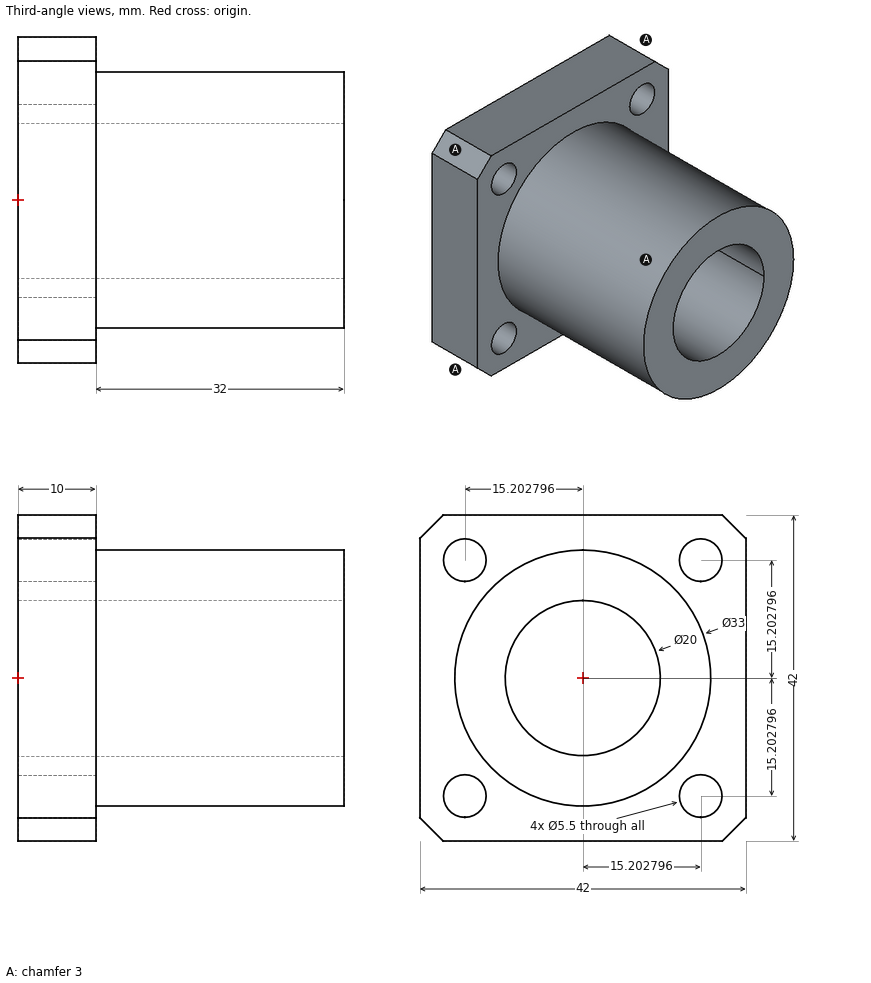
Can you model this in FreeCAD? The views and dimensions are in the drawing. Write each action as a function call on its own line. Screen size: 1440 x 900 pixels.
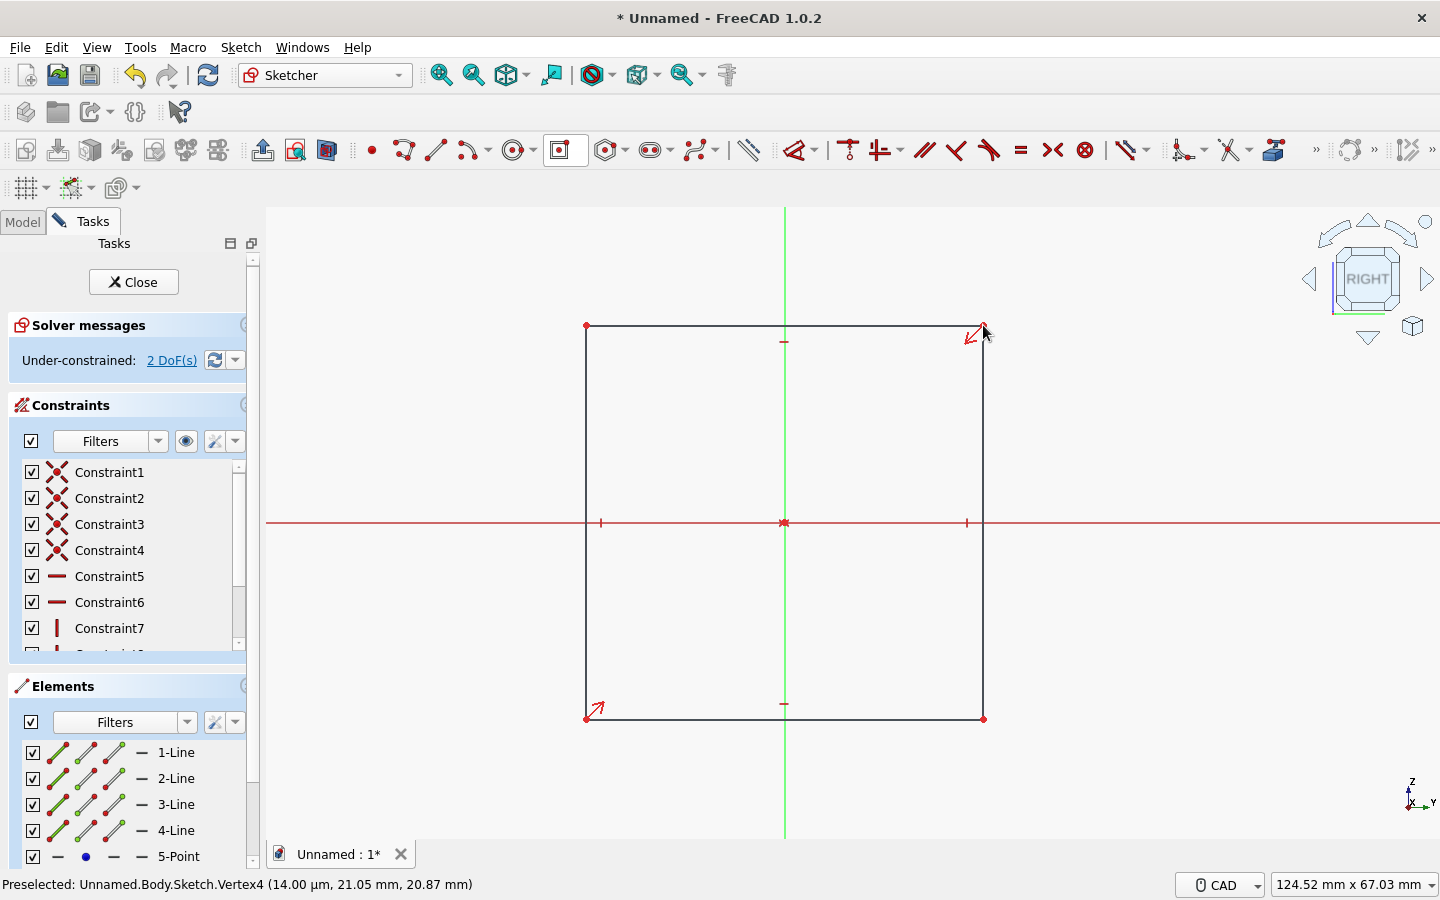
click(794, 150)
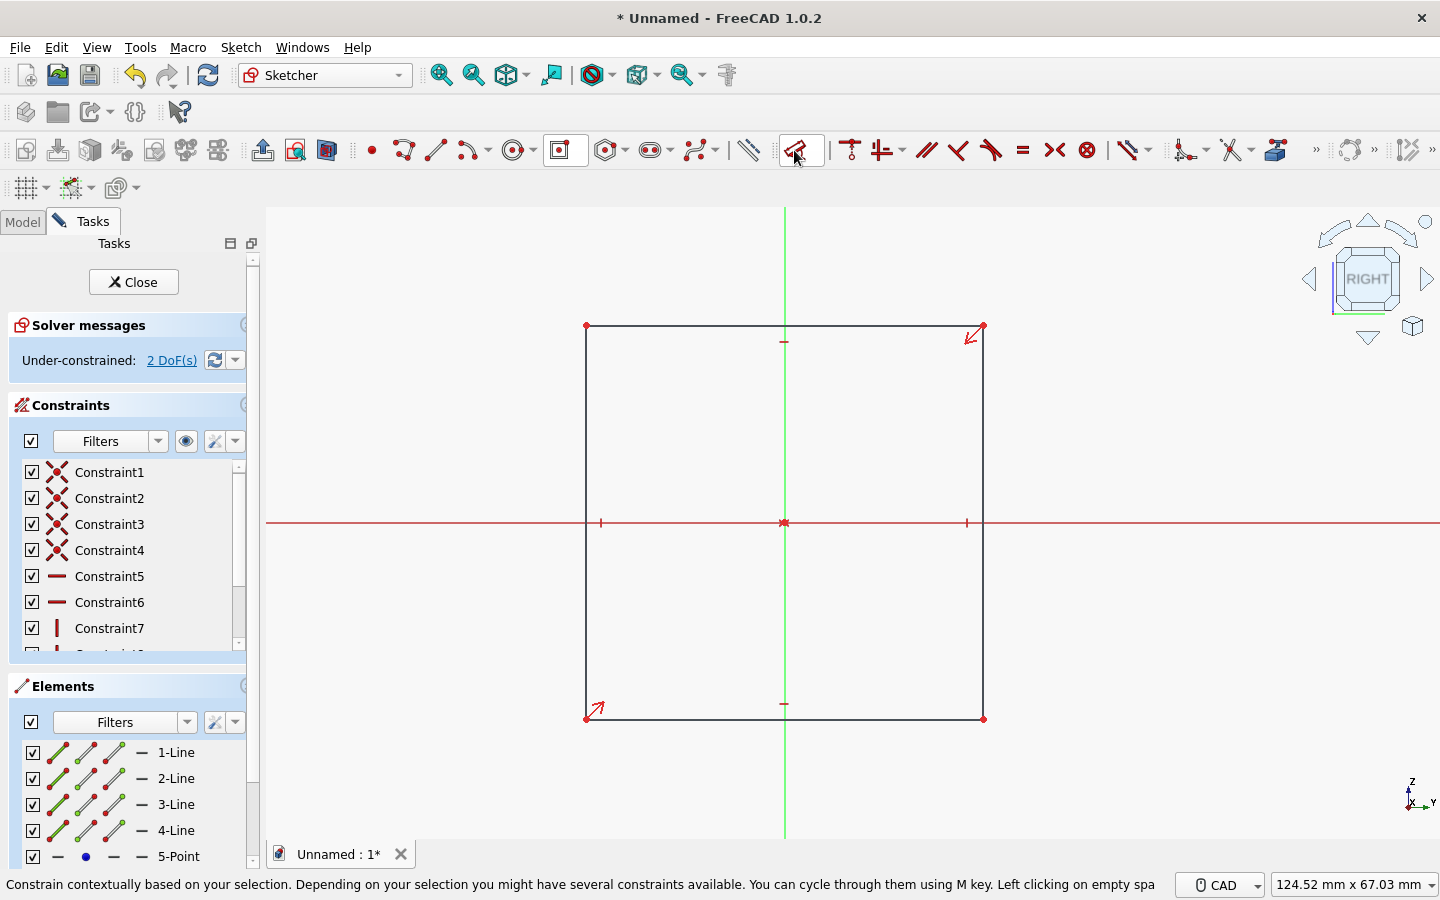
click(705, 720)
click(693, 754)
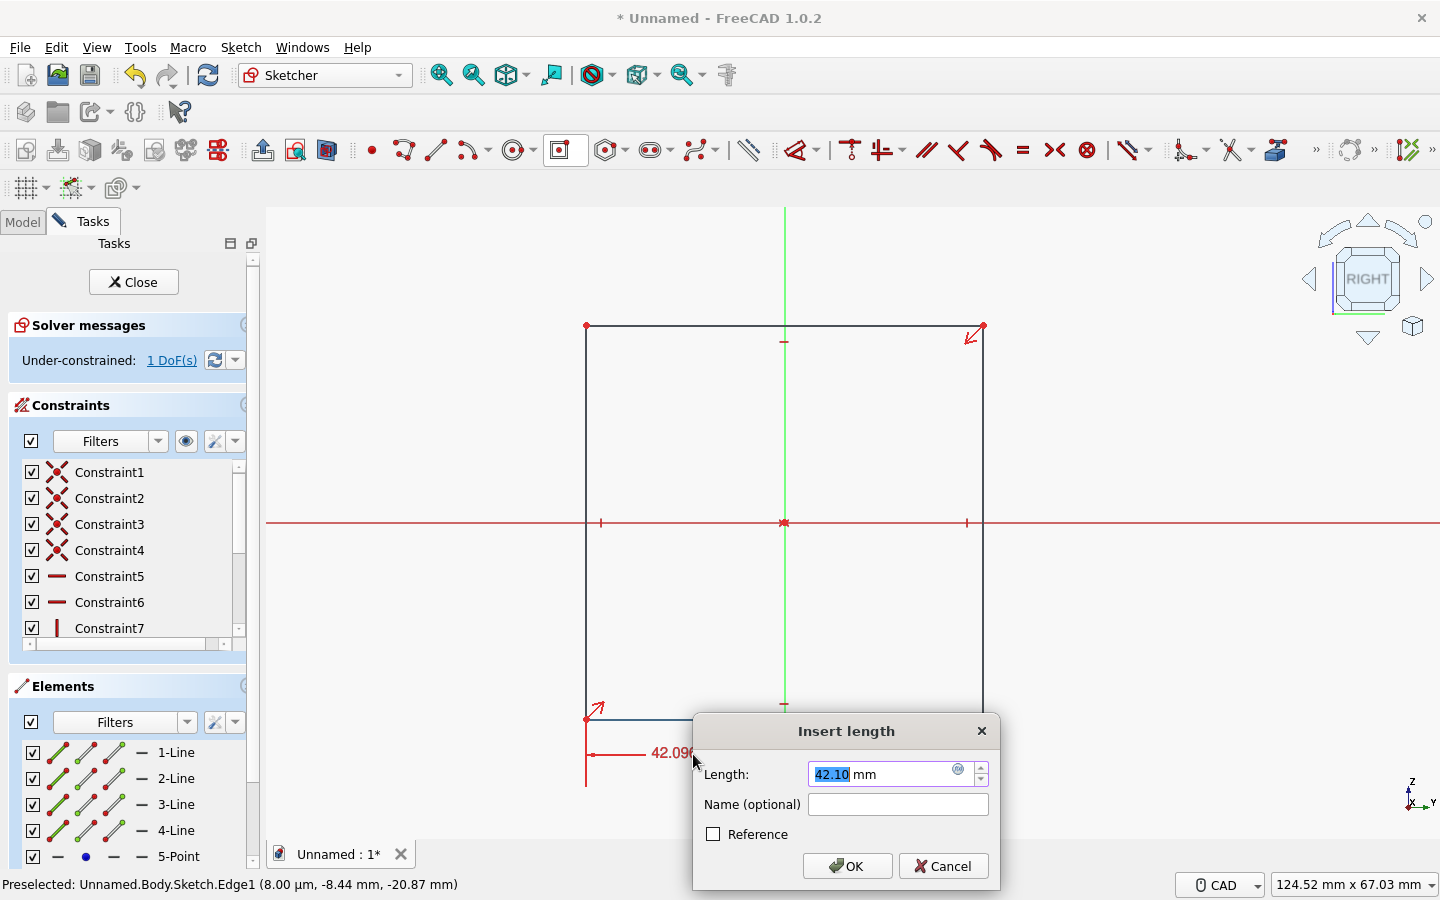
text(42)
key(Return)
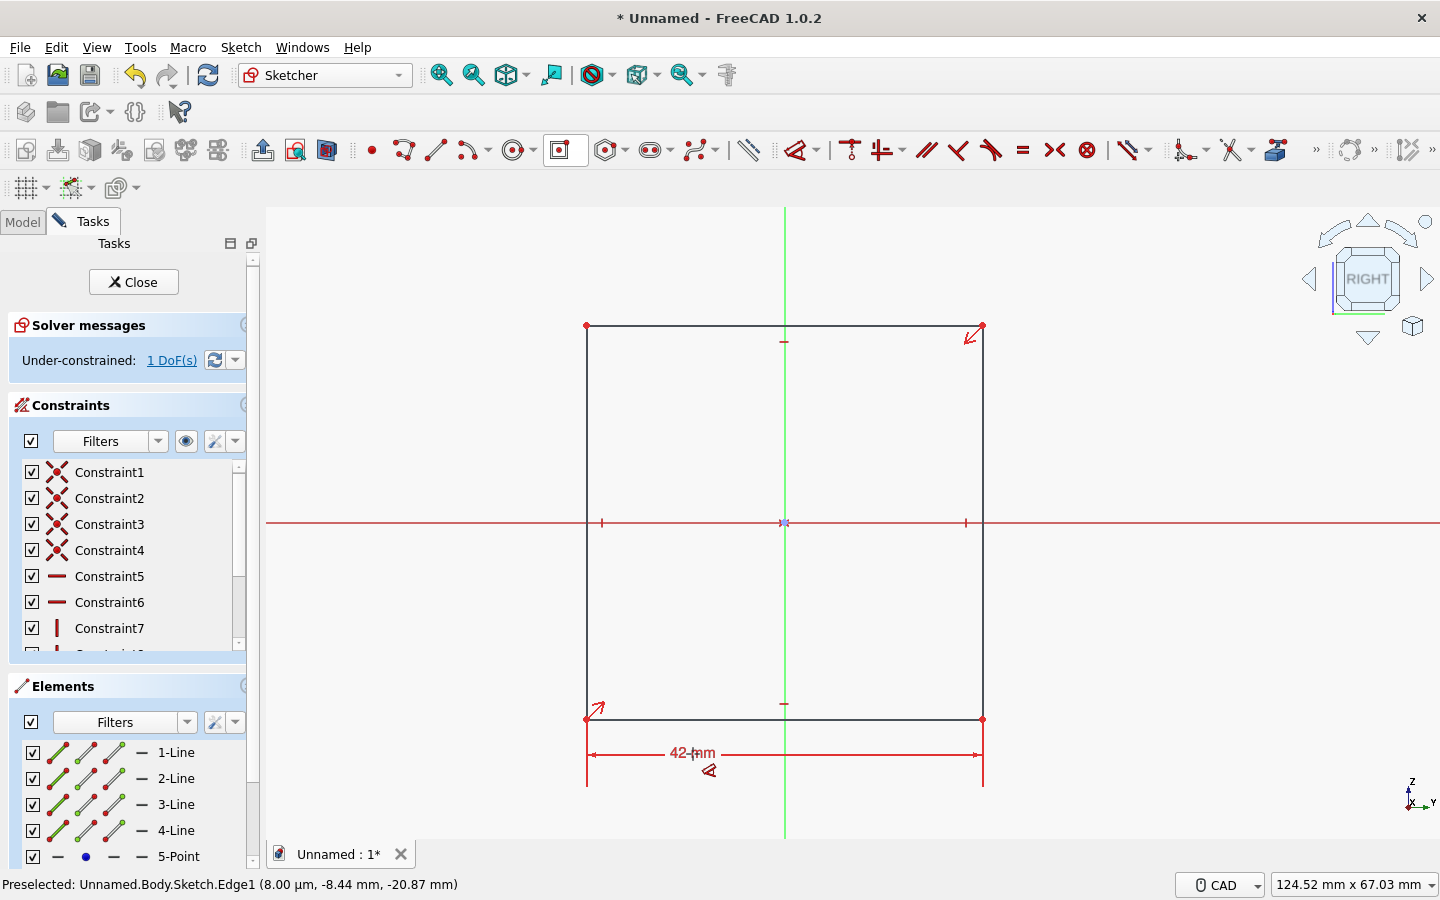
click(983, 601)
click(1017, 432)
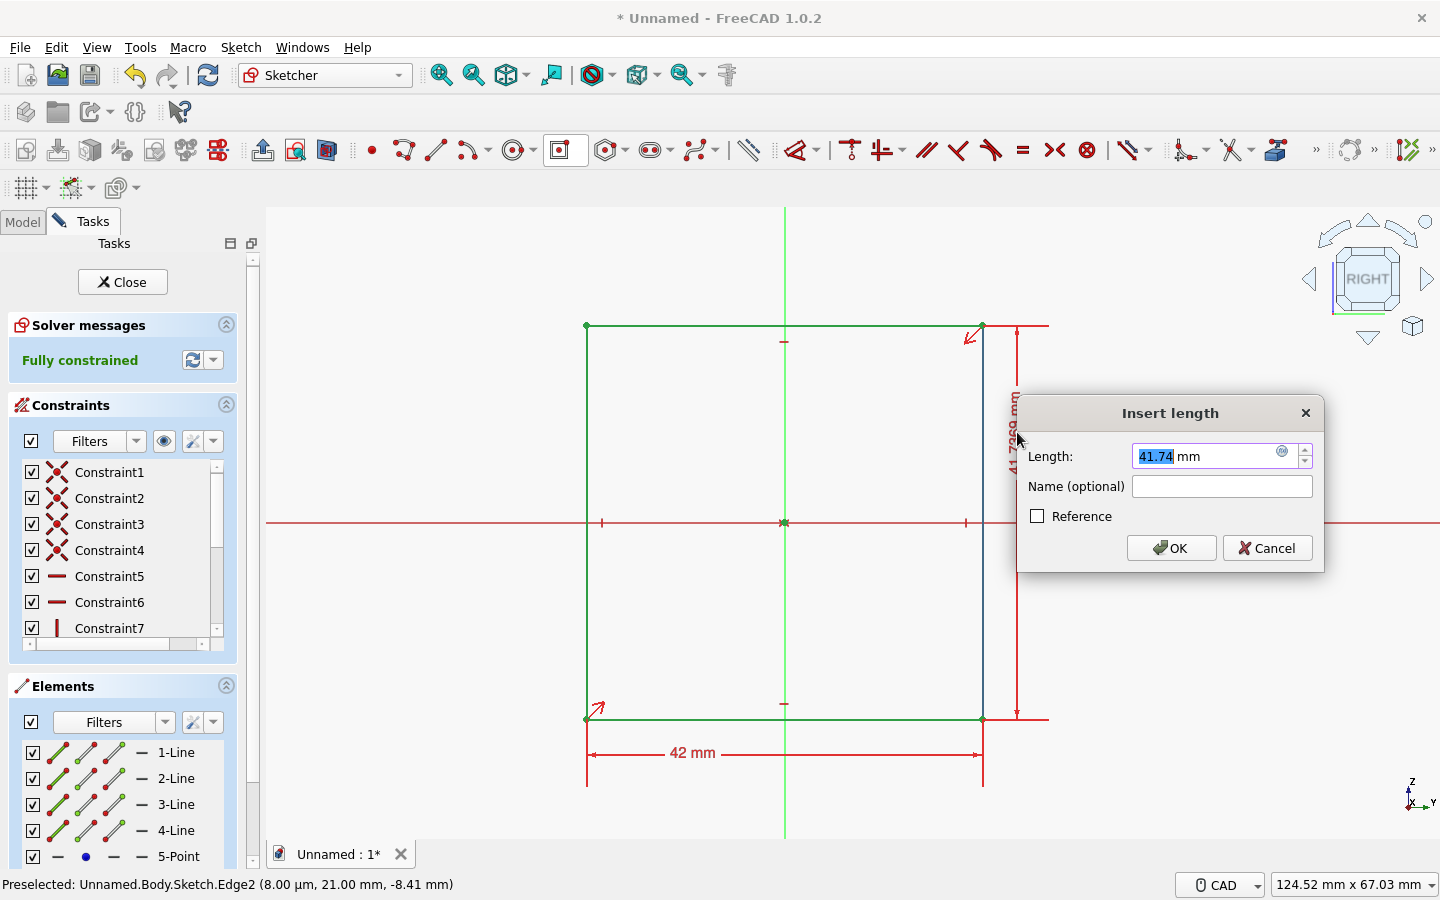
text(42)
key(Return)
key(Escape)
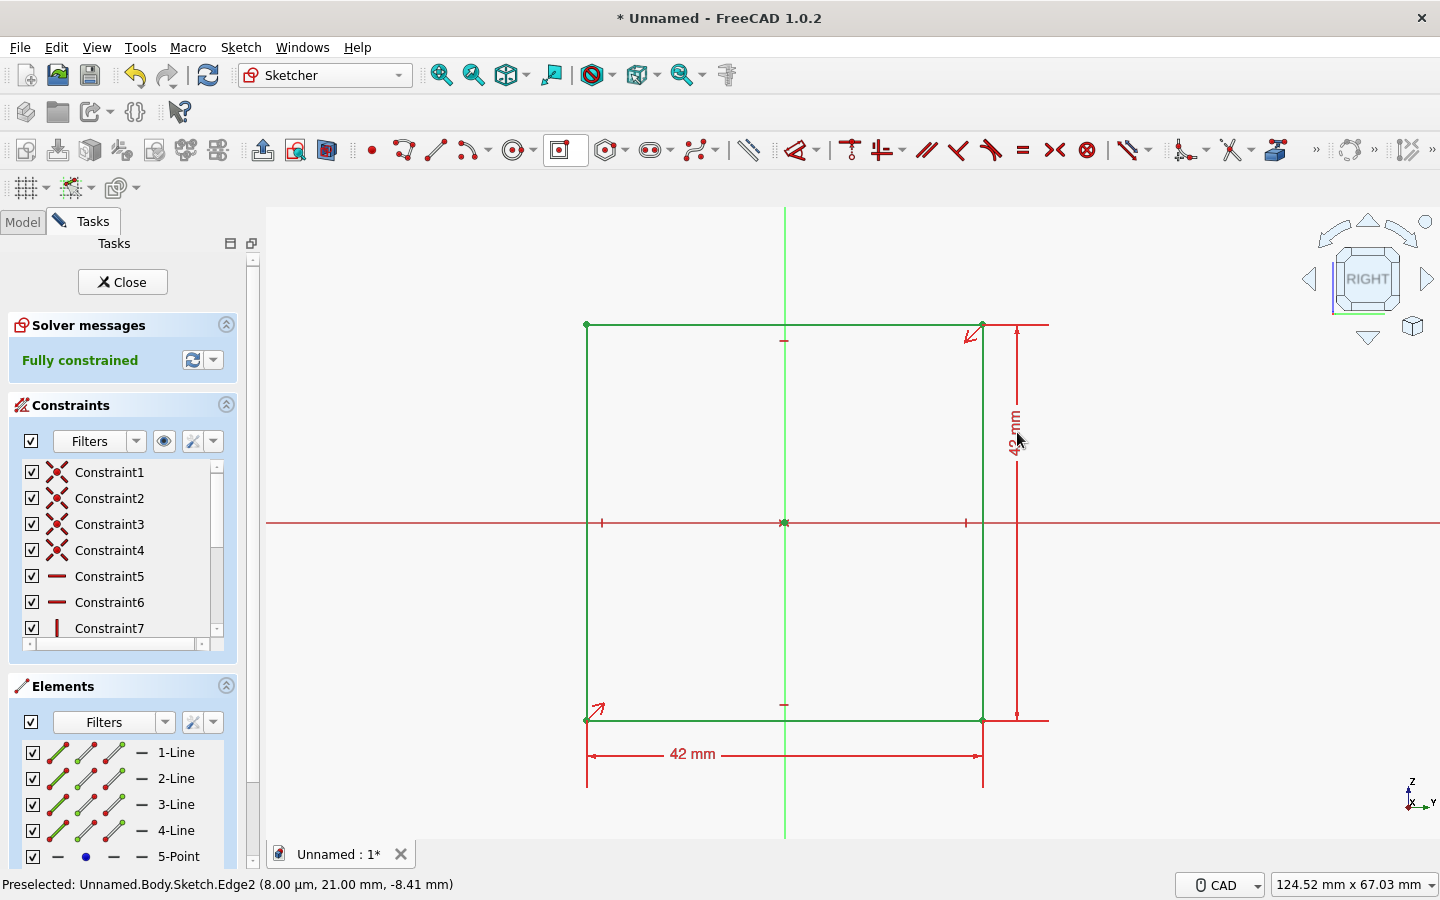
click(123, 282)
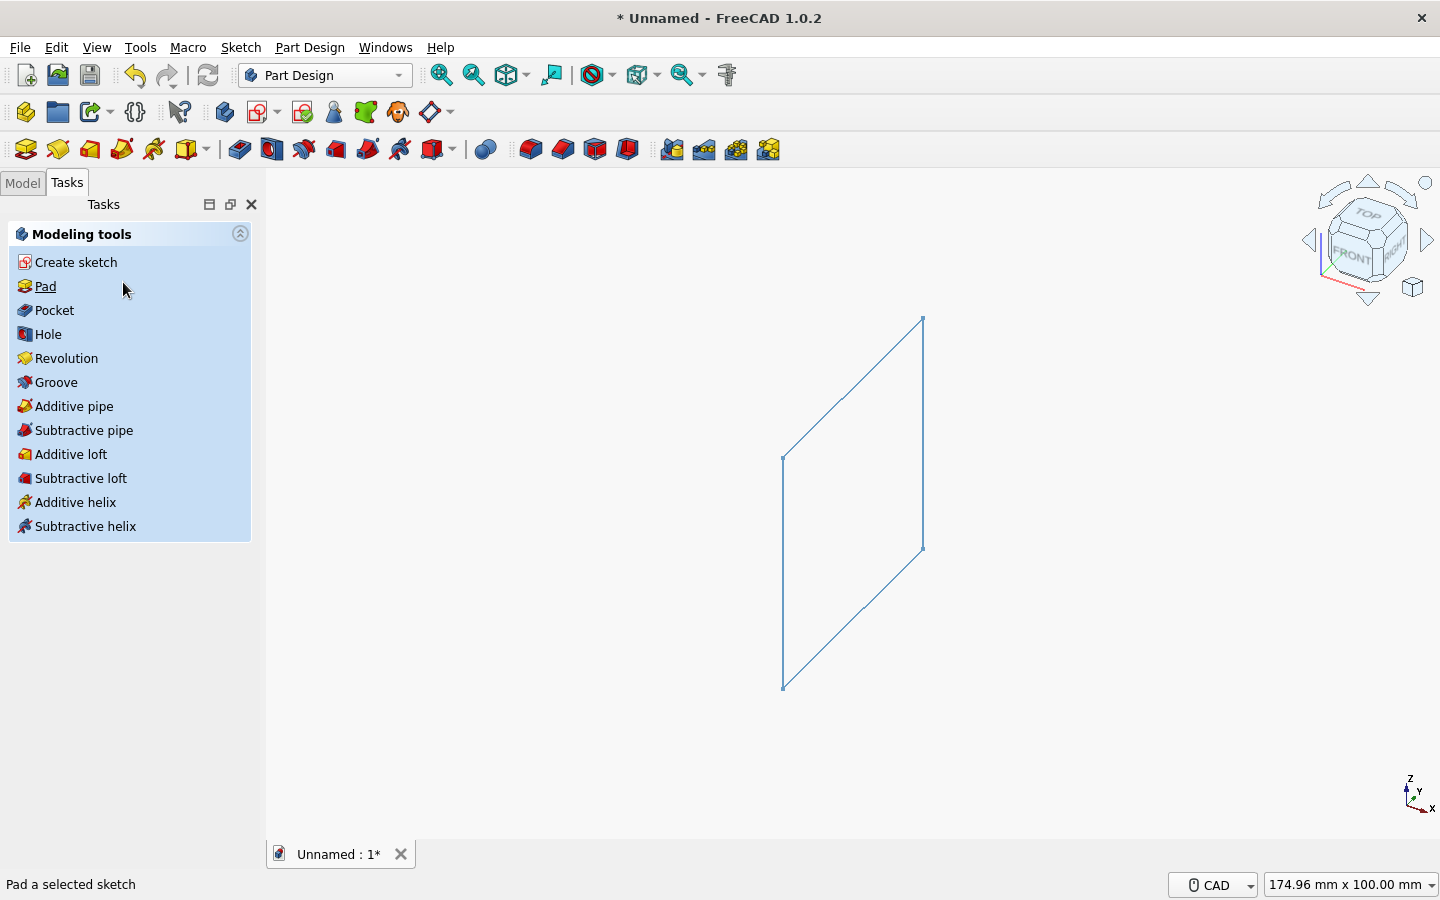
click(26, 150)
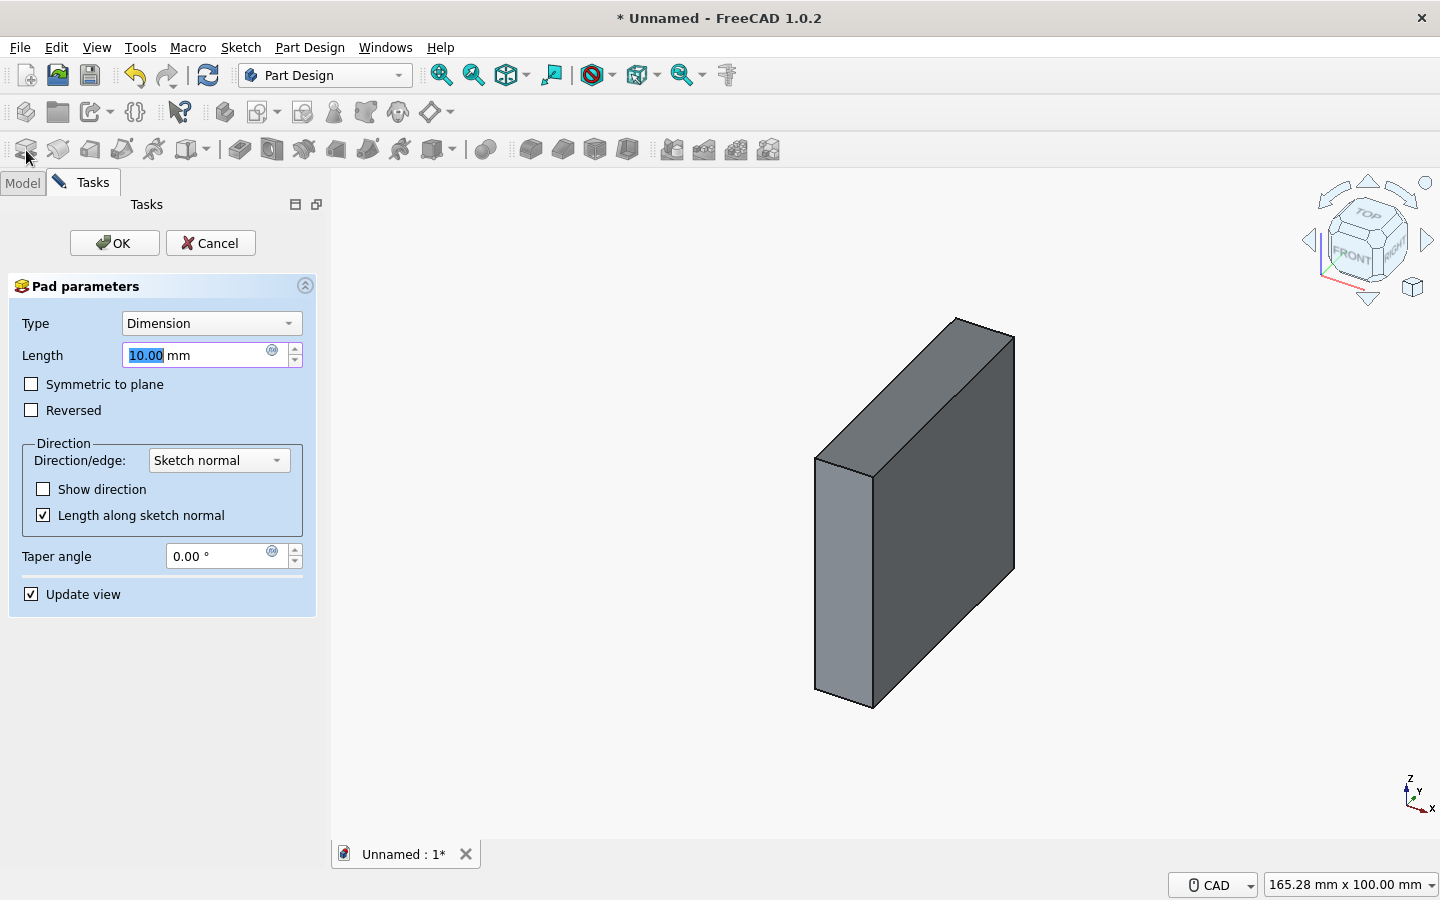
text(10)
key(Tab)